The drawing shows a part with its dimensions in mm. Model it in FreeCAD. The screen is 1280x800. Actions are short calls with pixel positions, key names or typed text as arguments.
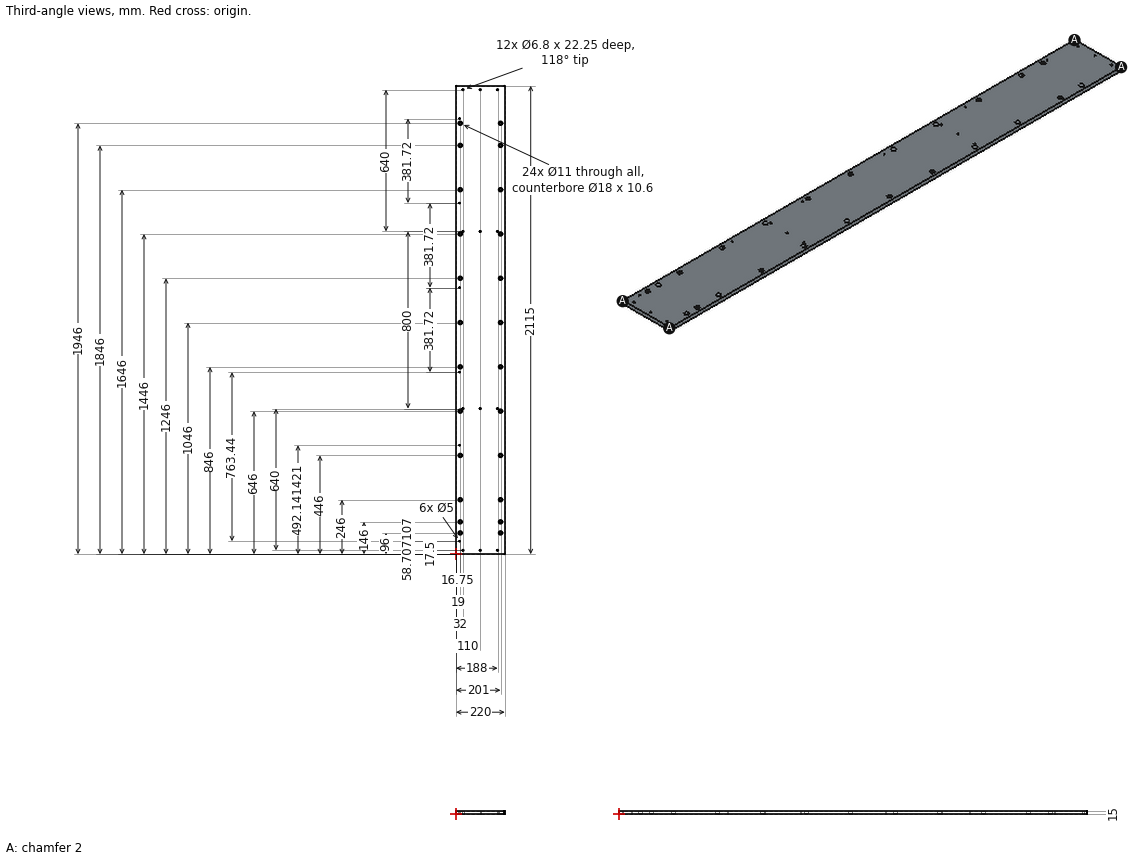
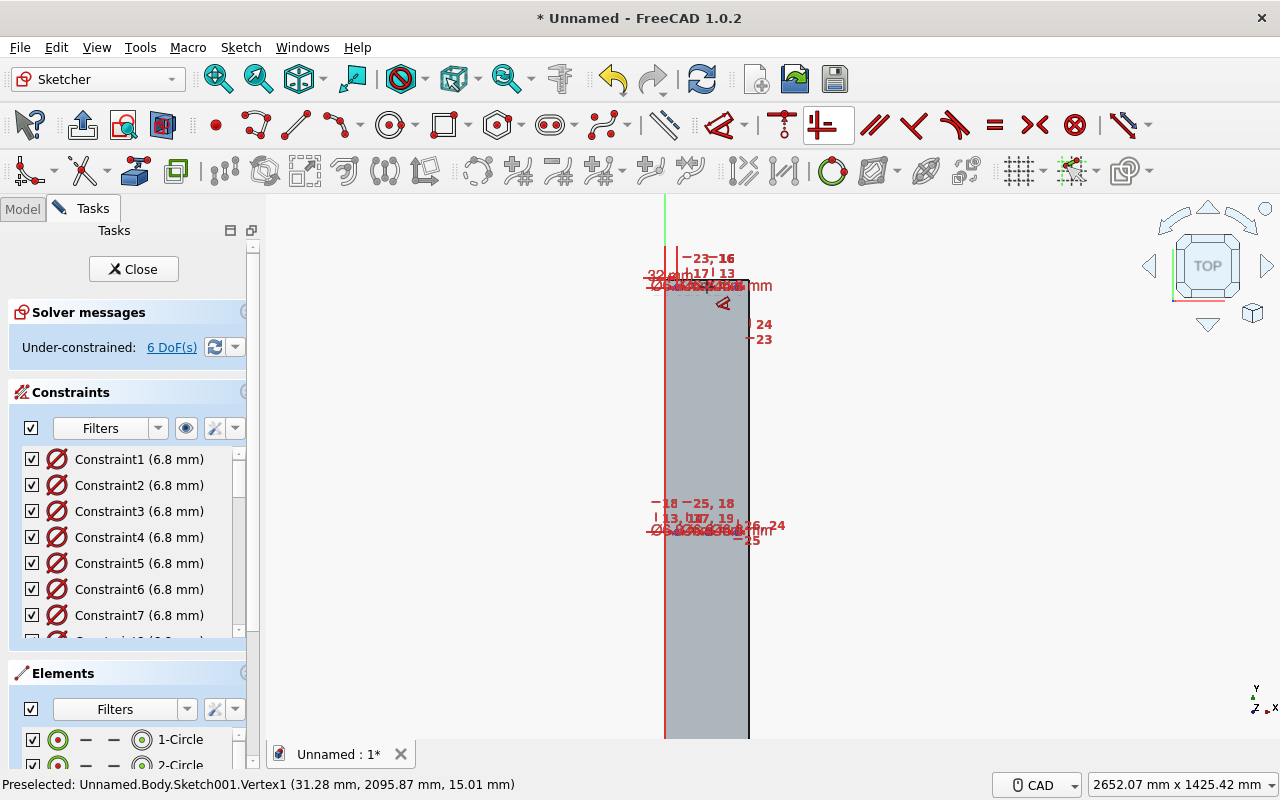
click(707, 288)
click(686, 254)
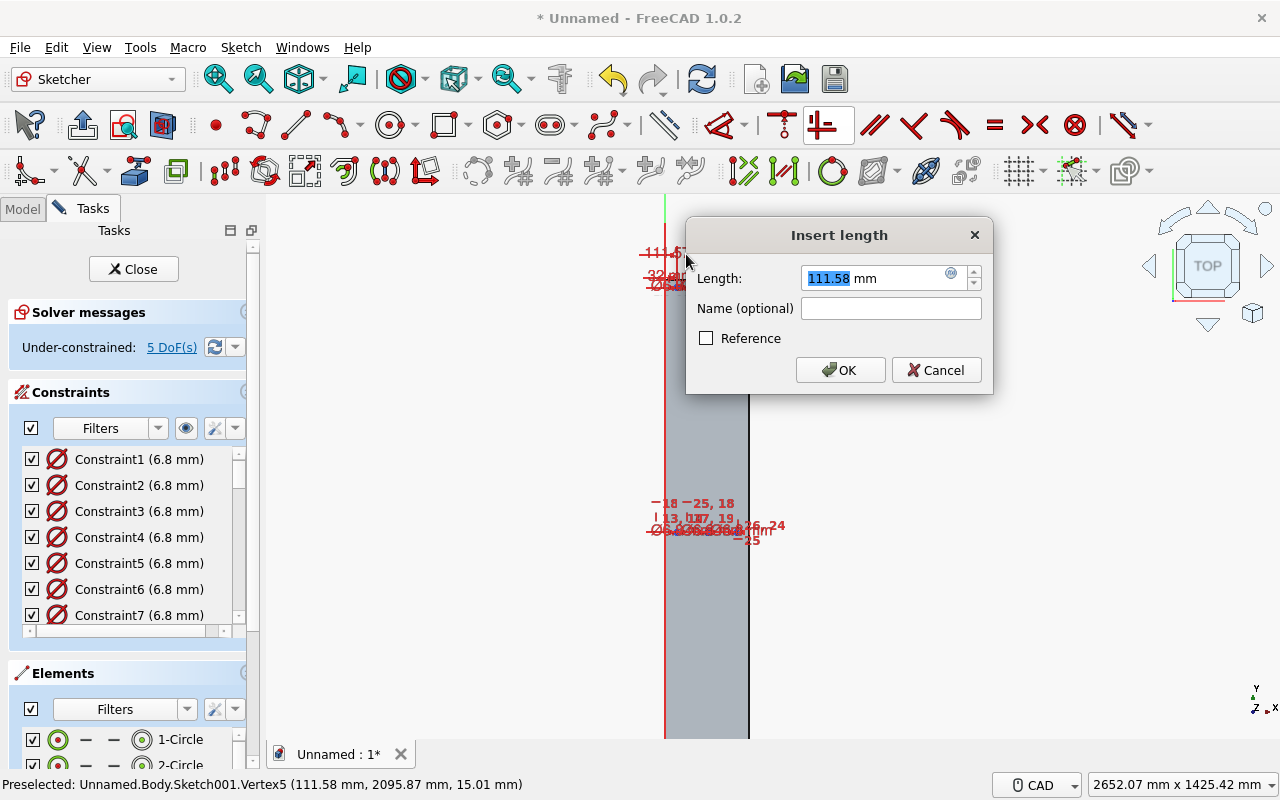
text(110)
key(Return)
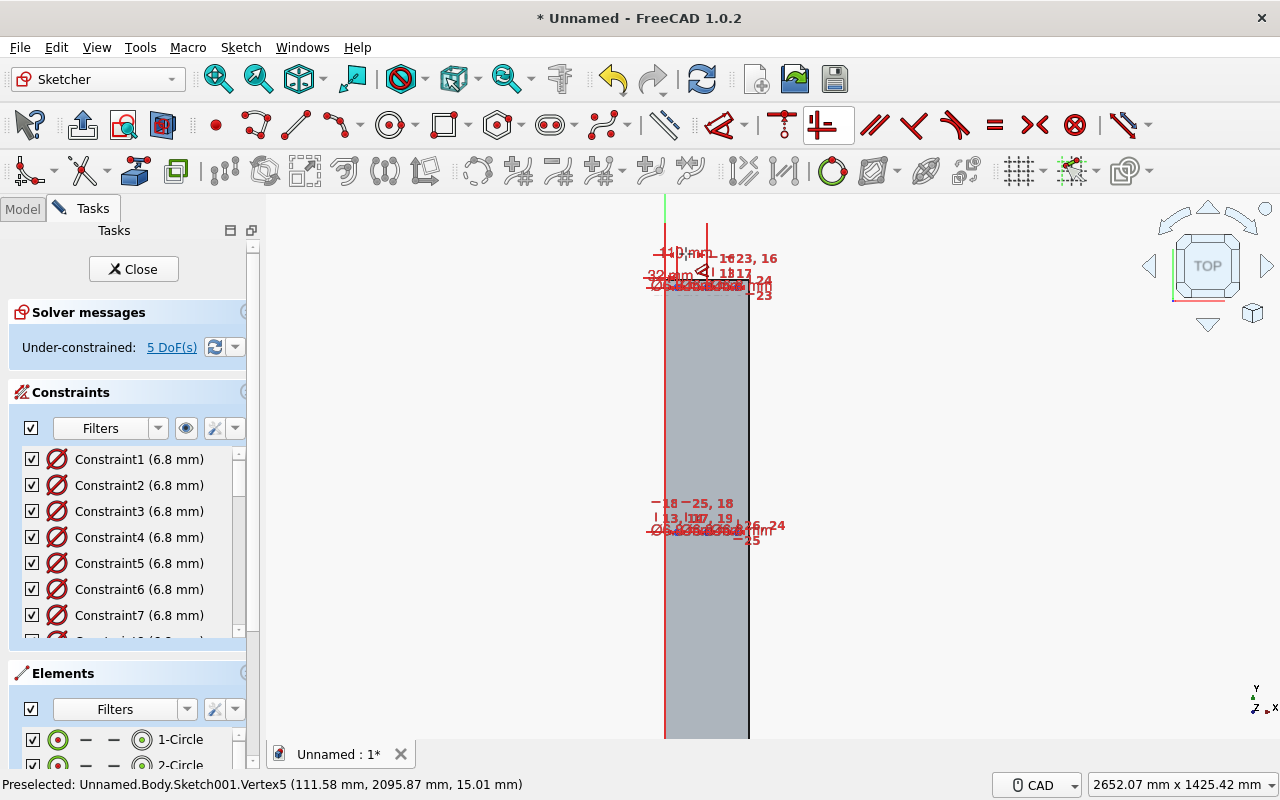
click(737, 288)
click(701, 230)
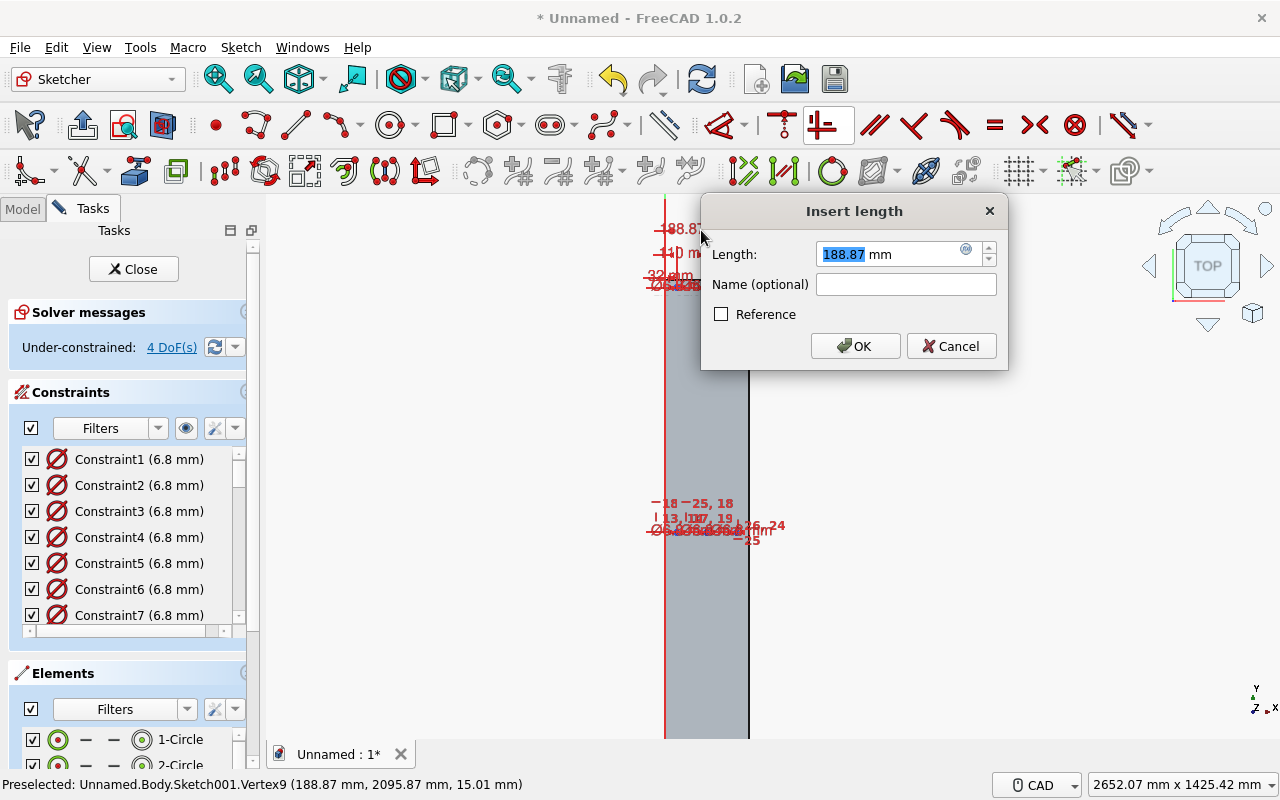
text(188)
key(Return)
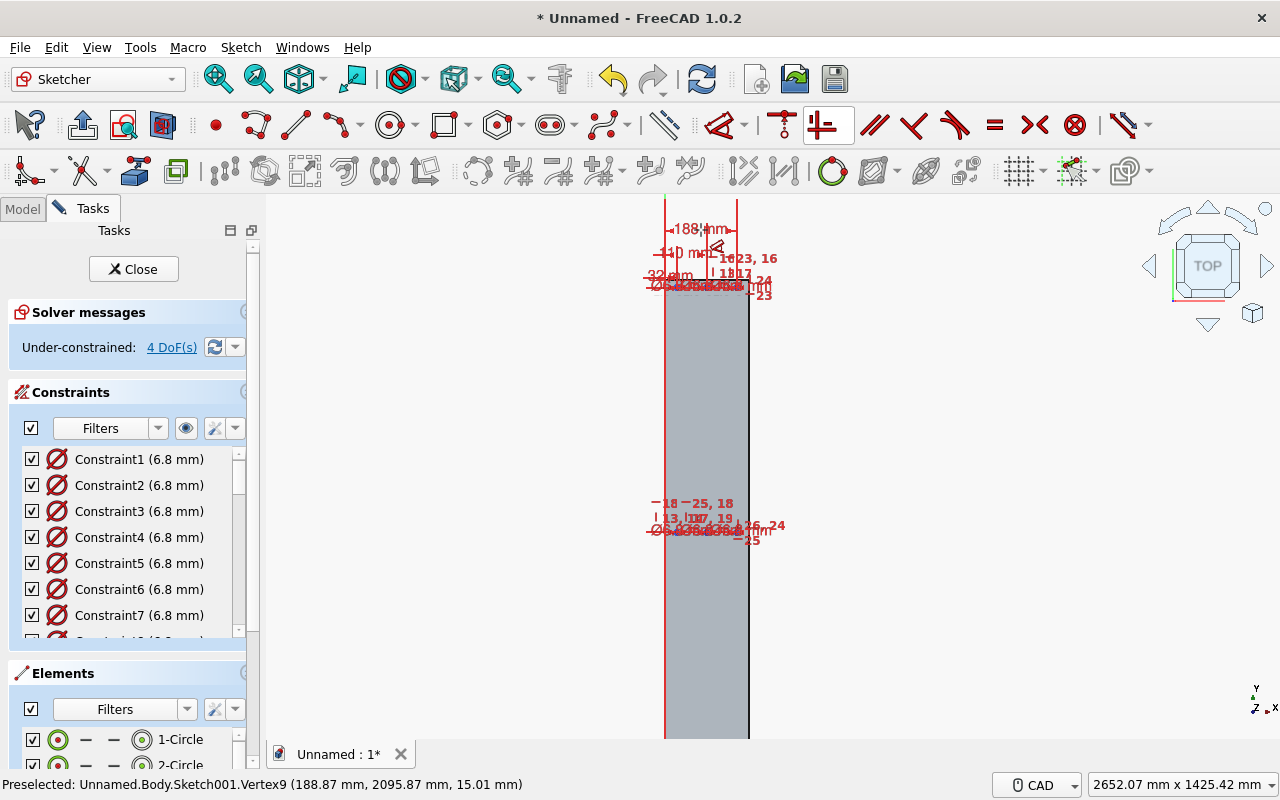
scroll(707, 286, down, 4)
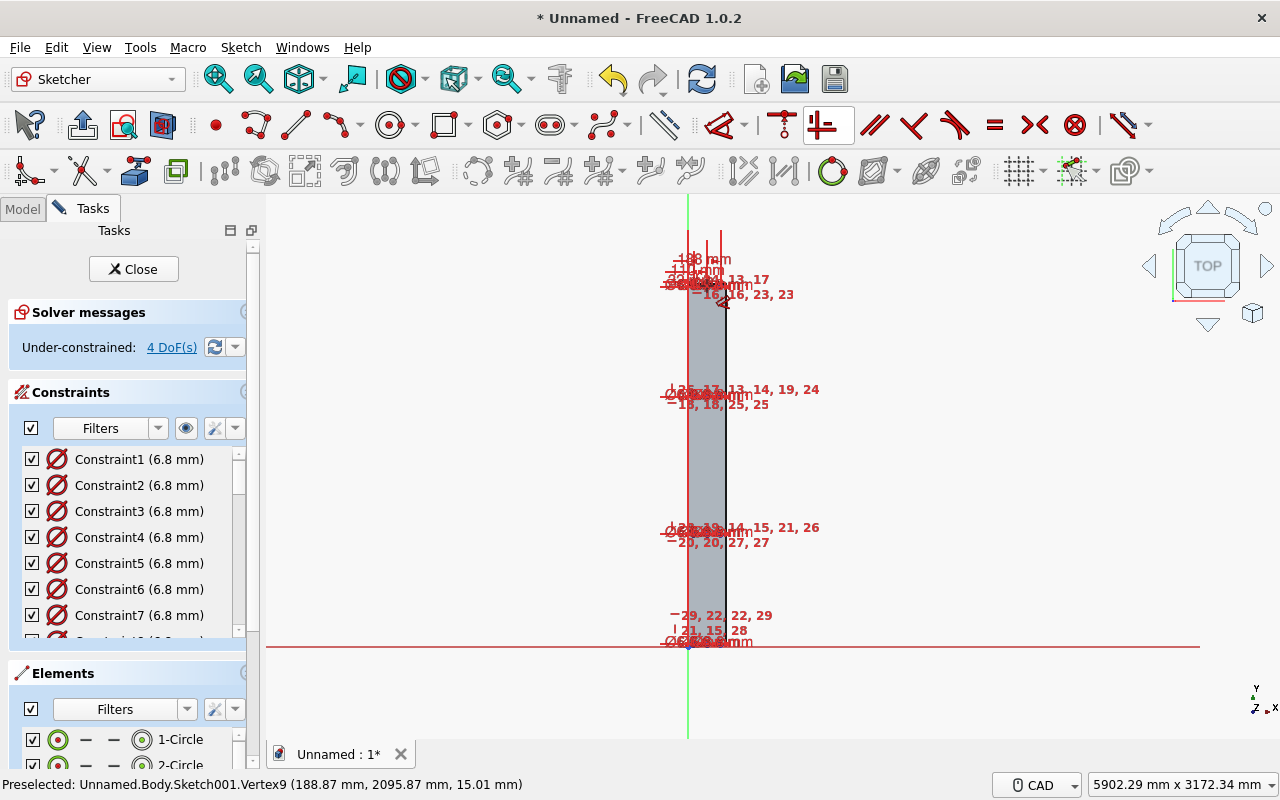
scroll(694, 644, up, 13)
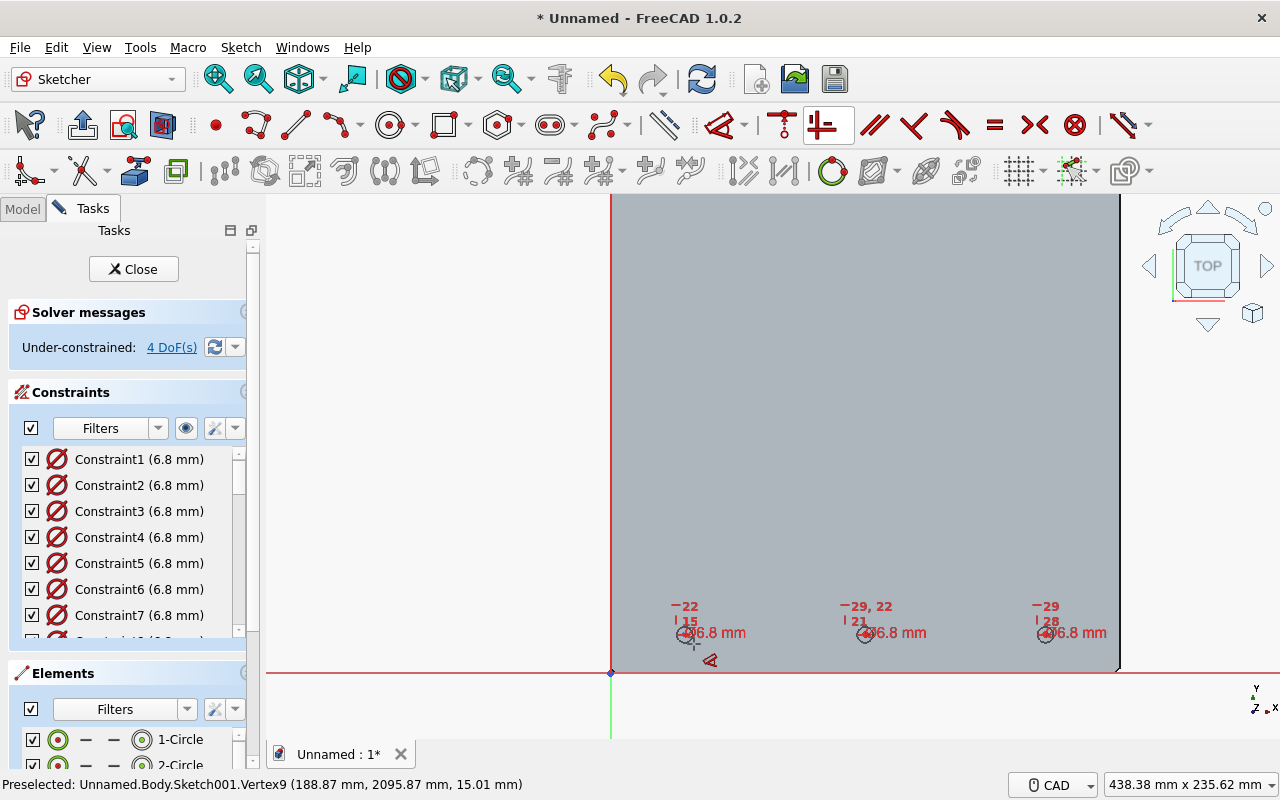
click(685, 635)
click(577, 654)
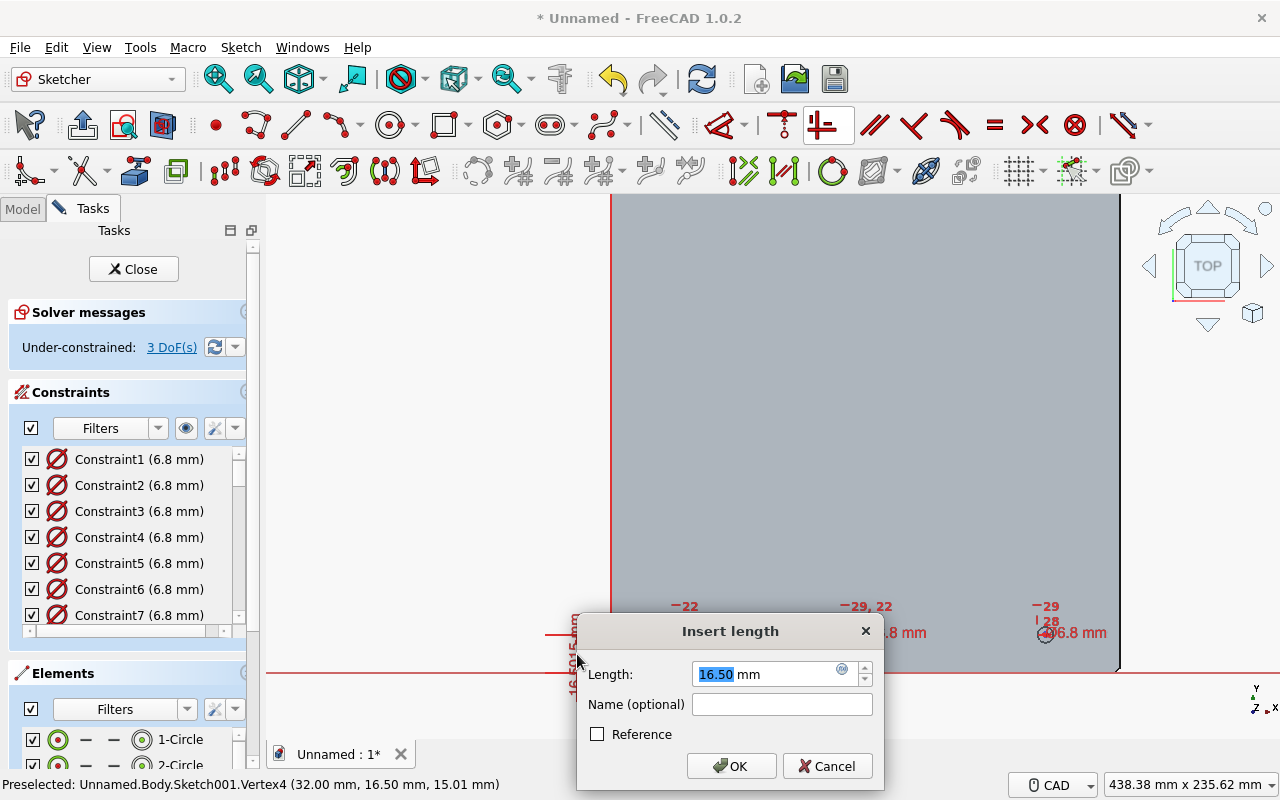
text(17.5)
key(Return)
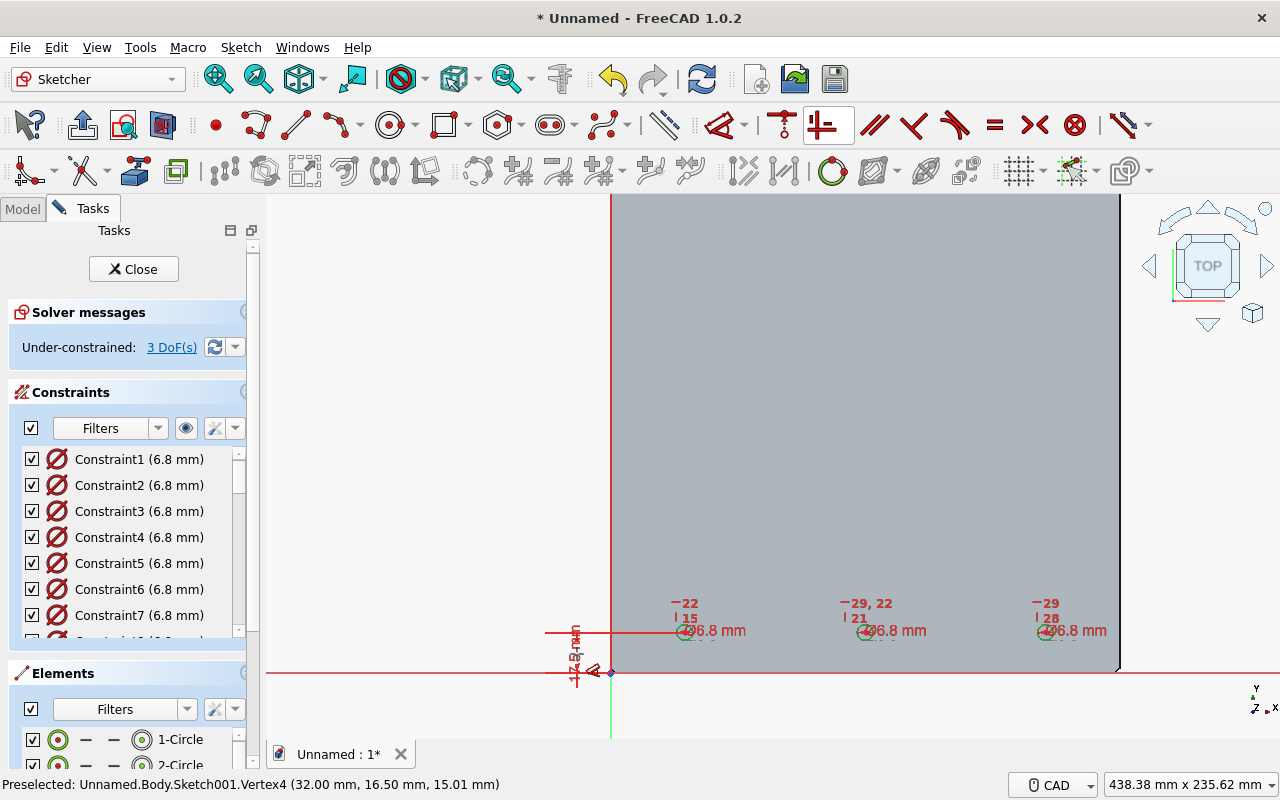
scroll(694, 645, down, 13)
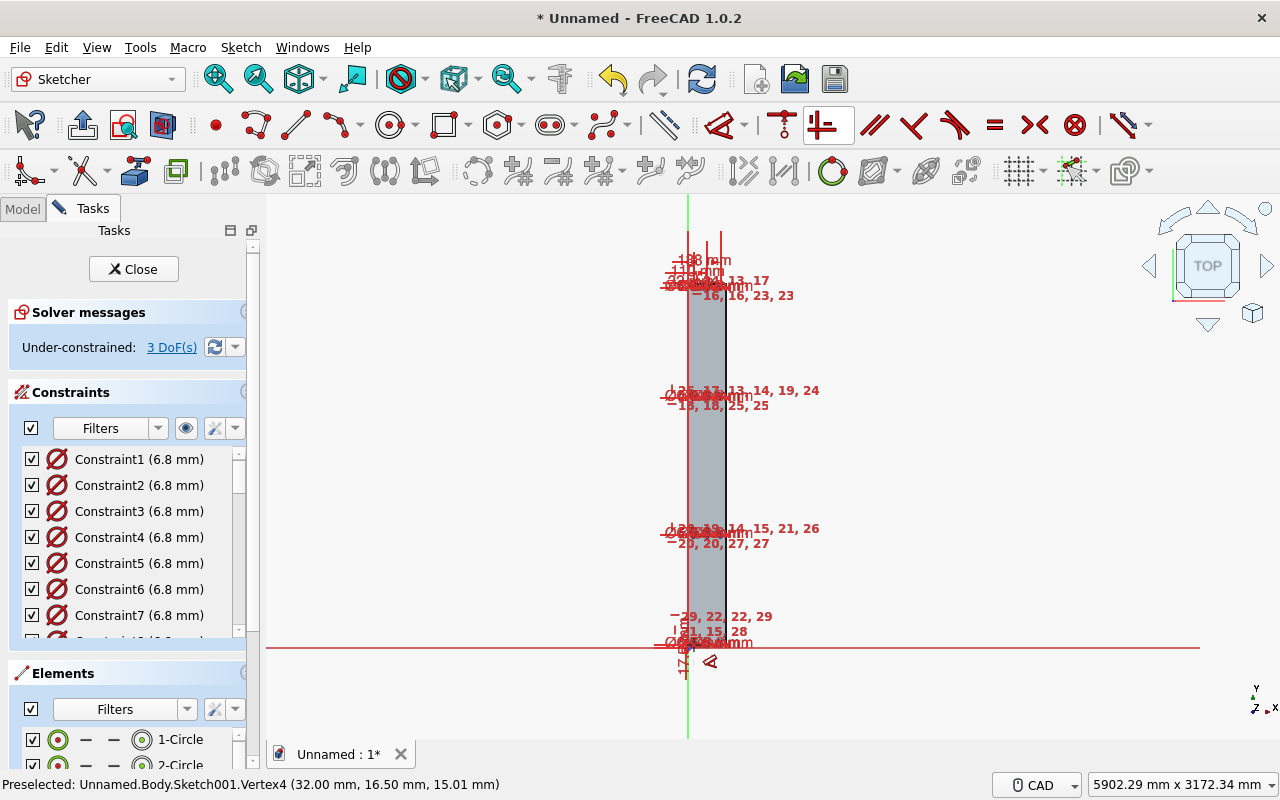
click(694, 288)